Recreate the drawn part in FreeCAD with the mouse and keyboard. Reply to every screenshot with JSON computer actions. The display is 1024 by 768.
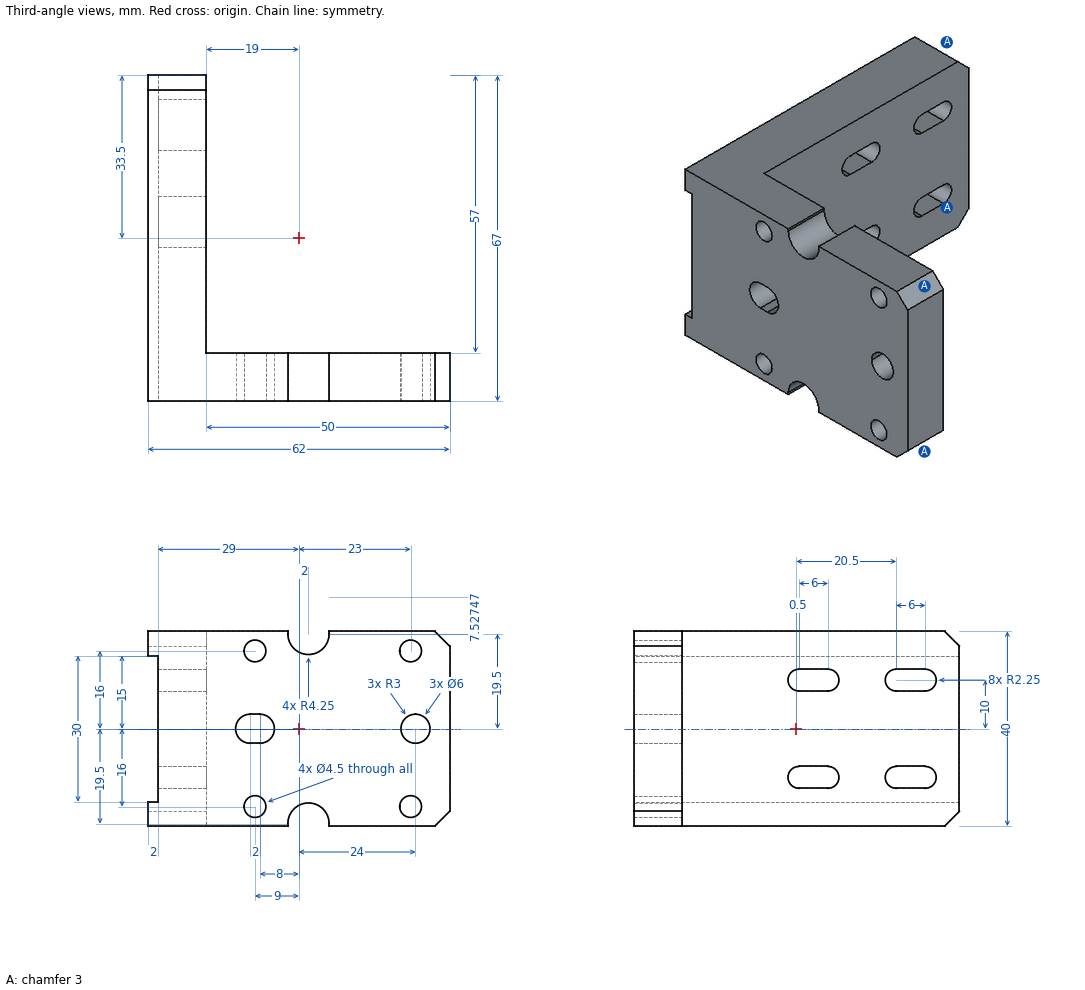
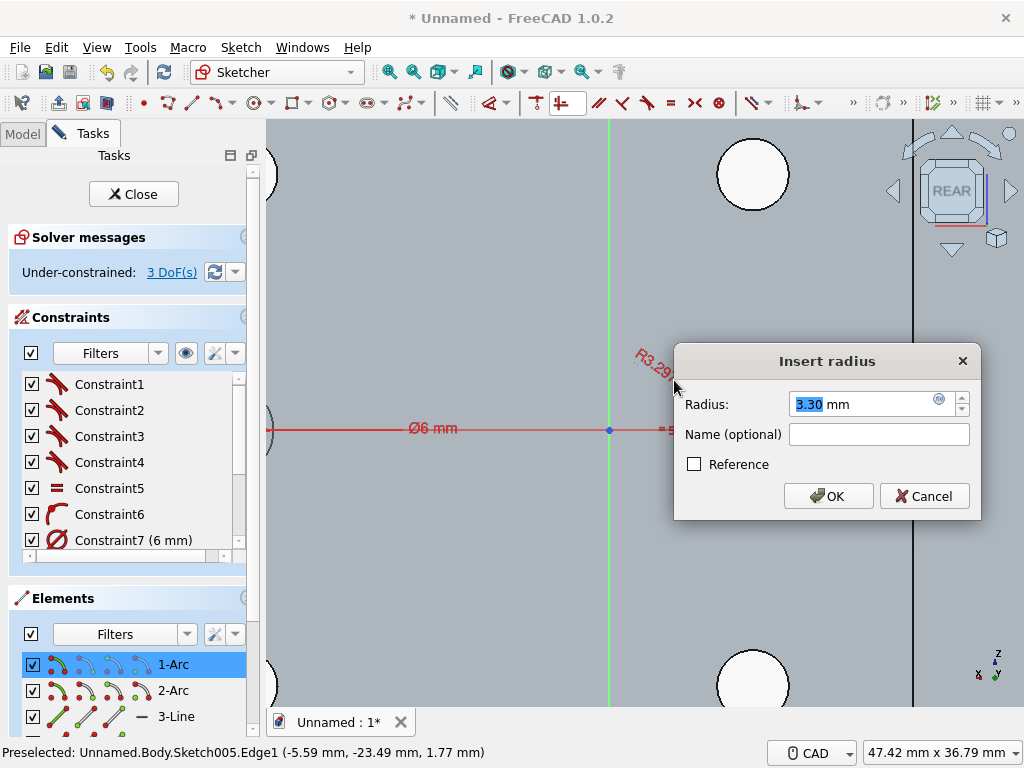
{"action": "type", "text": "3"}
{"action": "key", "text": "Return"}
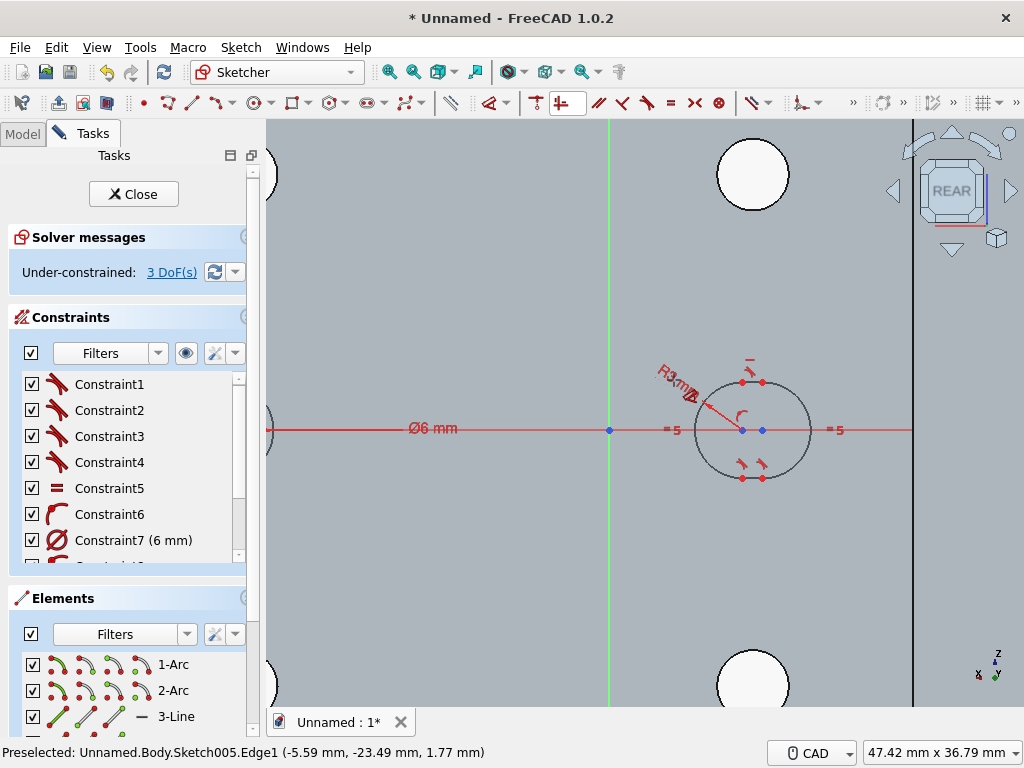
{"action": "scroll", "coordinate": [753, 382], "scroll_direction": "up", "scroll_amount": 2}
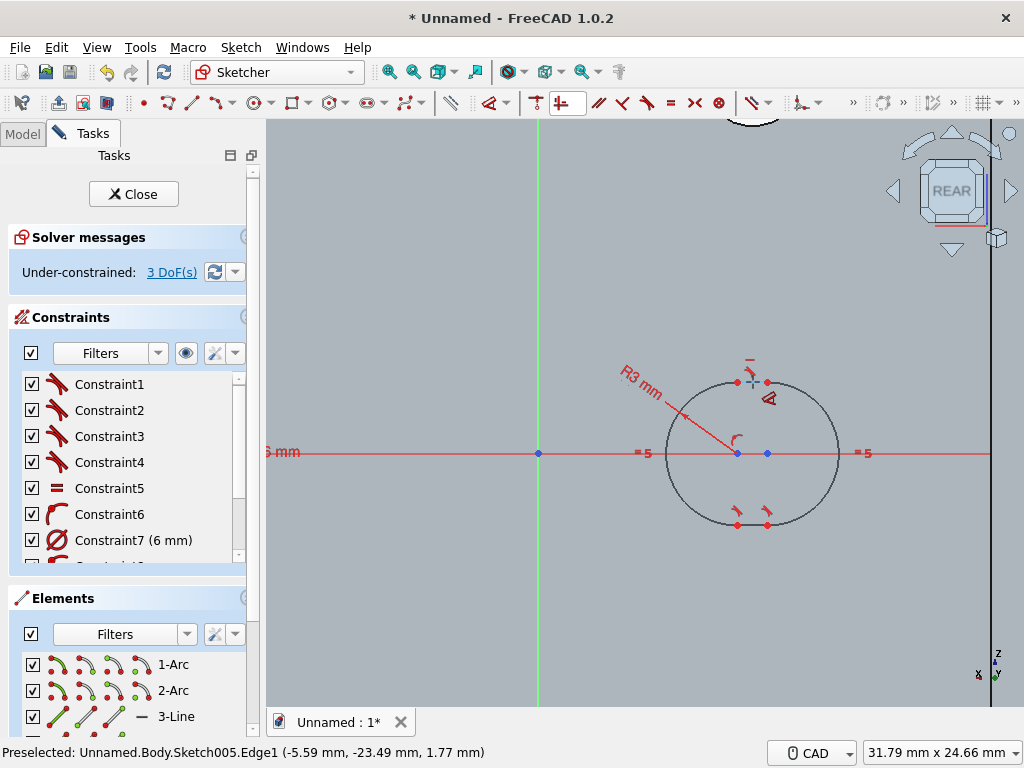
{"action": "left_click", "coordinate": [752, 382]}
{"action": "left_click", "coordinate": [752, 348]}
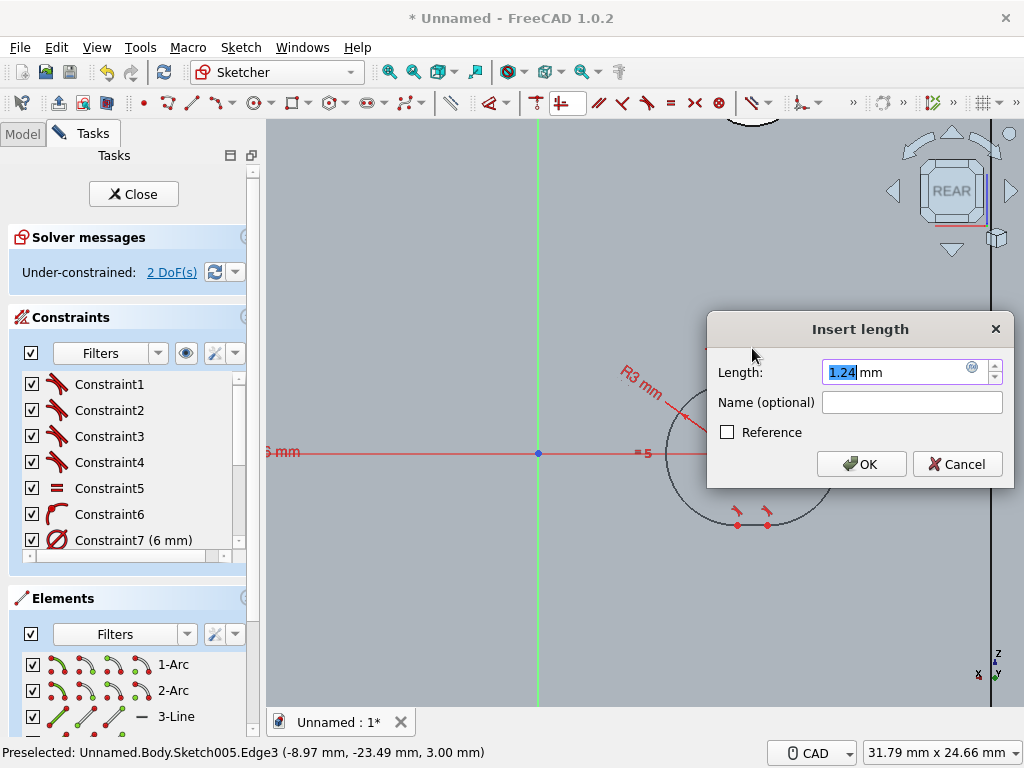
{"action": "type", "text": "2"}
{"action": "key", "text": "Return"}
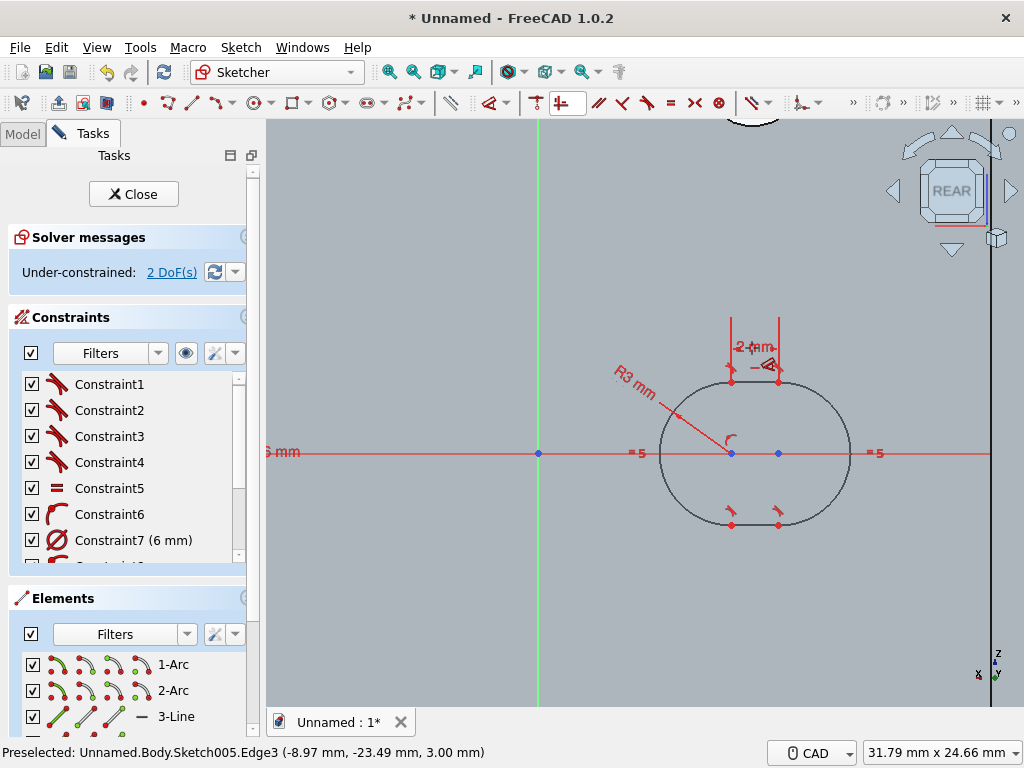
{"action": "left_click", "coordinate": [731, 382]}
{"action": "left_click", "coordinate": [635, 348]}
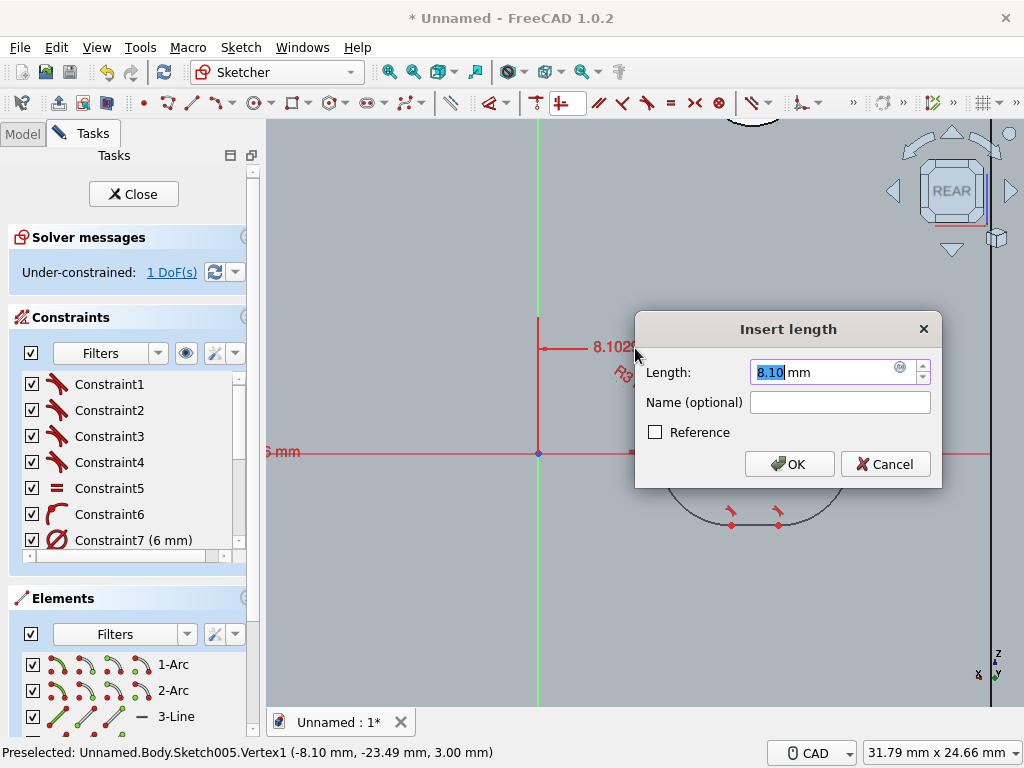
{"action": "type", "text": "8"}
{"action": "key", "text": "Return"}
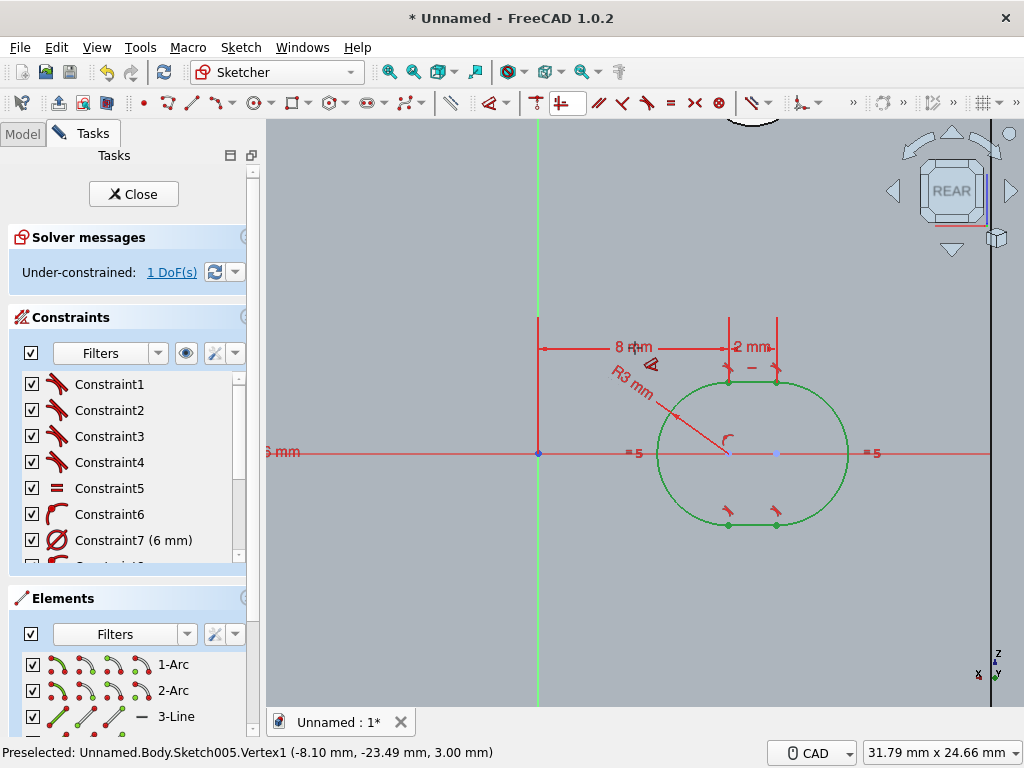
{"action": "scroll", "coordinate": [744, 380], "scroll_direction": "down", "scroll_amount": 4}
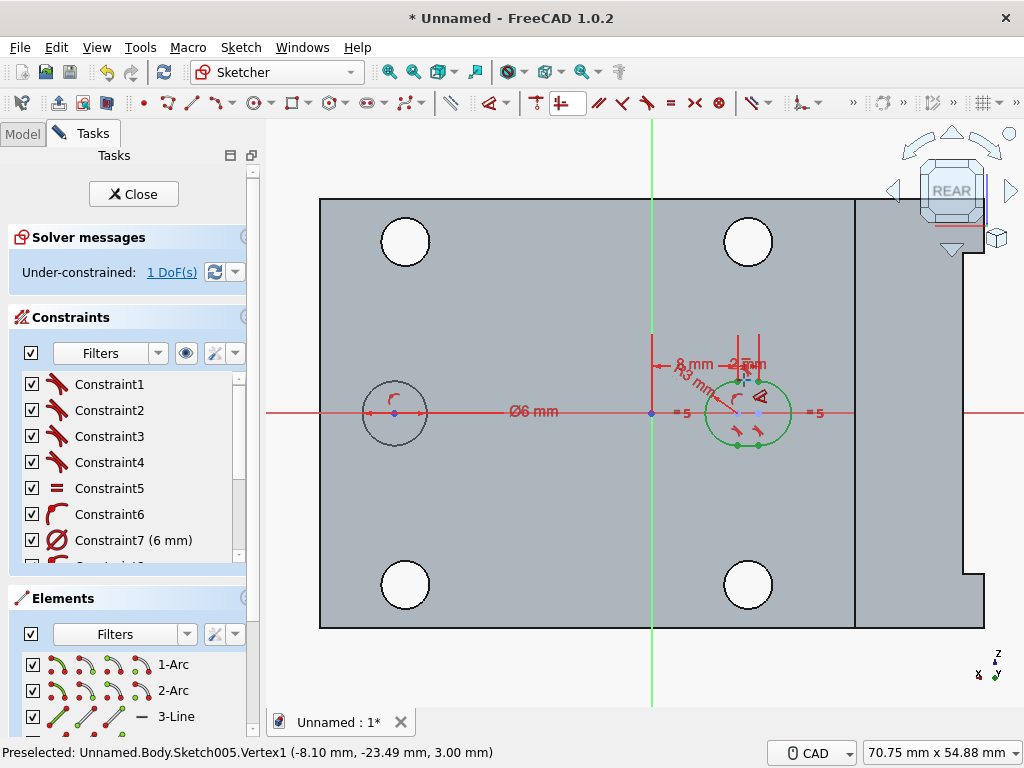
{"action": "left_click", "coordinate": [395, 413]}
{"action": "left_click", "coordinate": [523, 447]}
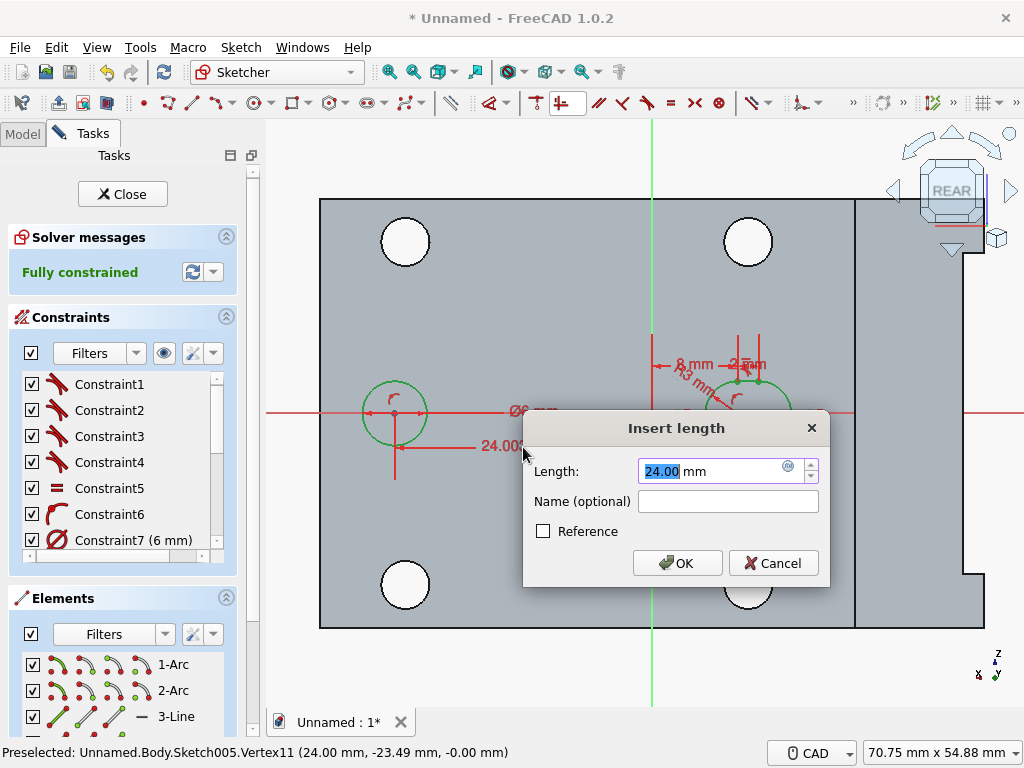
{"action": "type", "text": "24"}
{"action": "key", "text": "Return"}
{"action": "key", "text": "Escape"}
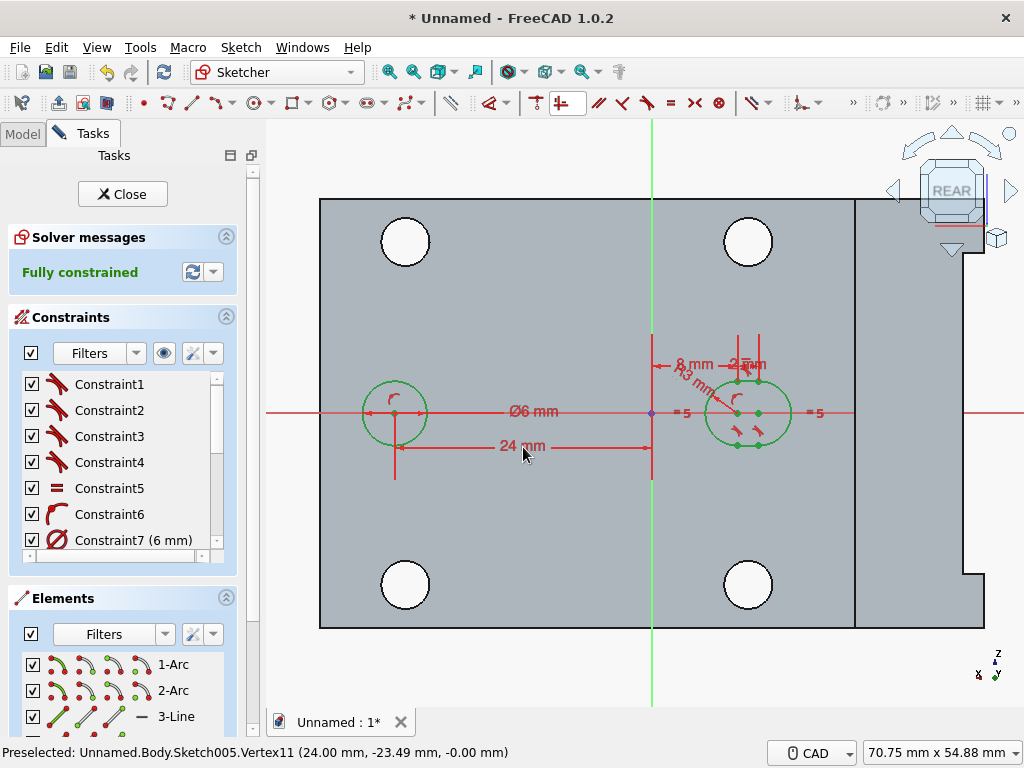
{"action": "left_click", "coordinate": [123, 194]}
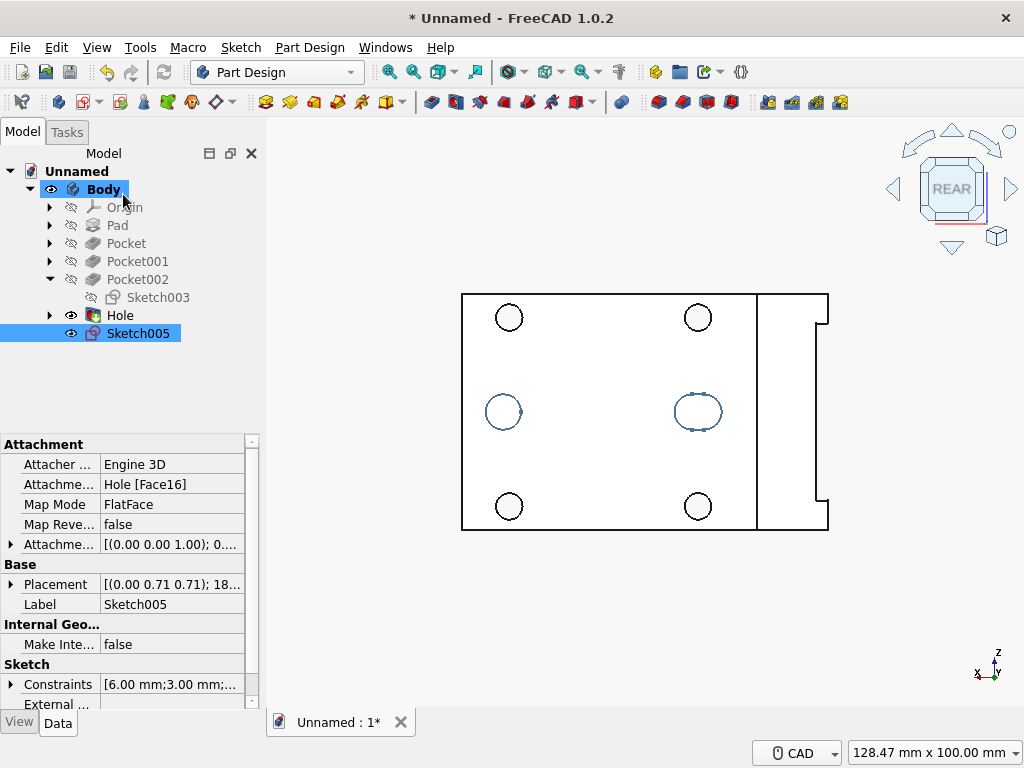
{"action": "left_click", "coordinate": [432, 102]}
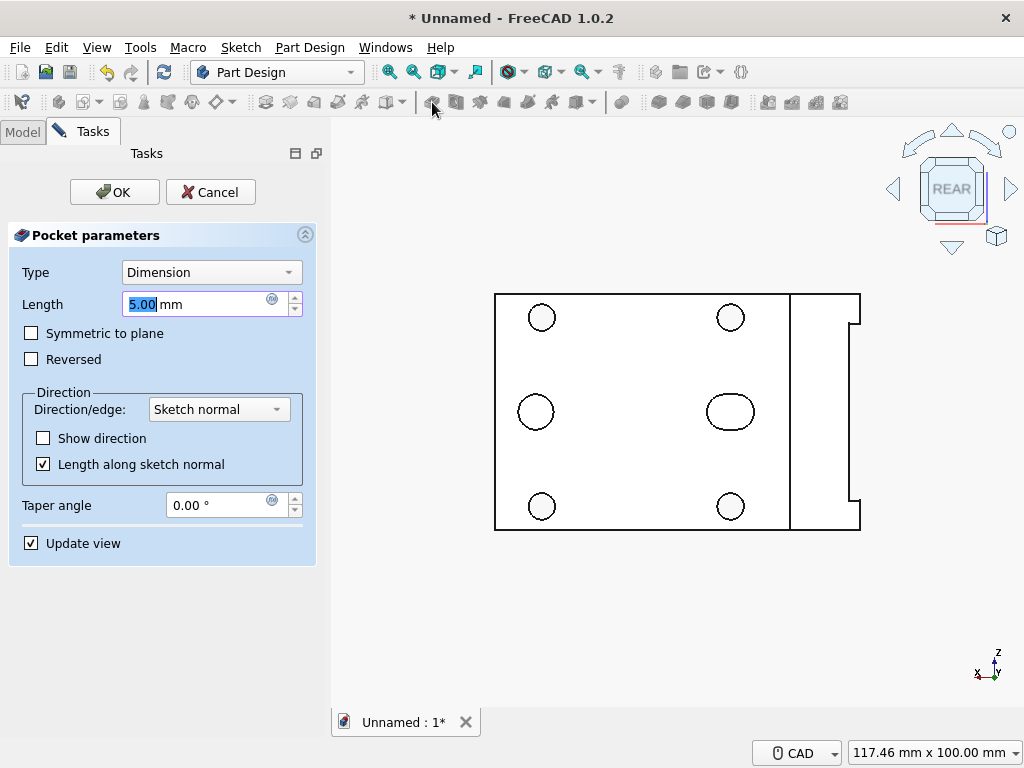
{"action": "left_click", "coordinate": [212, 272]}